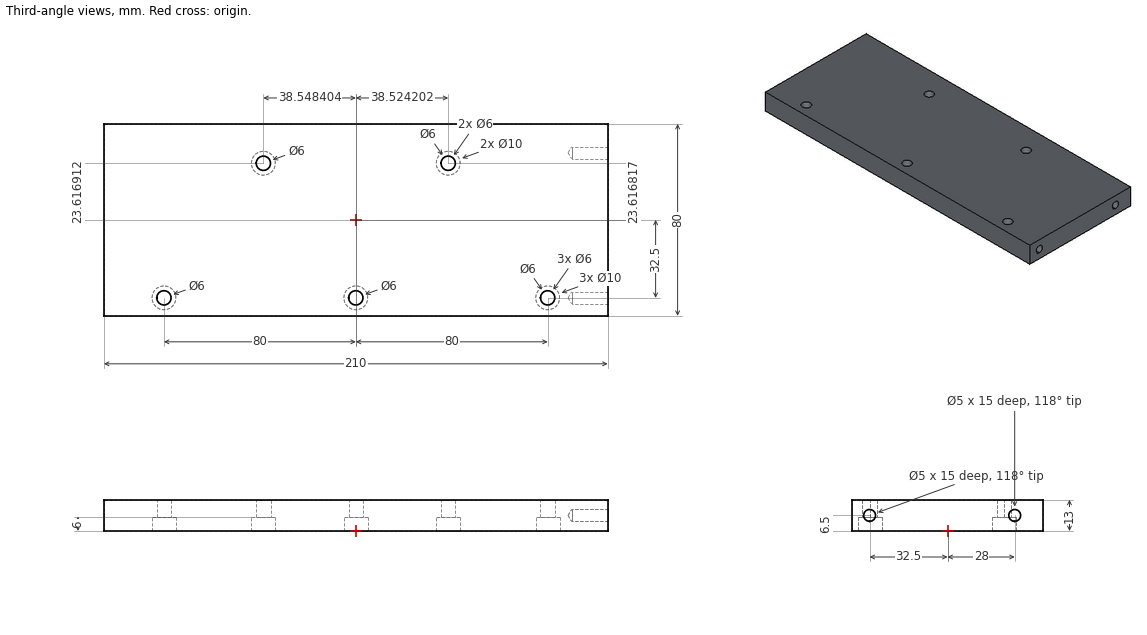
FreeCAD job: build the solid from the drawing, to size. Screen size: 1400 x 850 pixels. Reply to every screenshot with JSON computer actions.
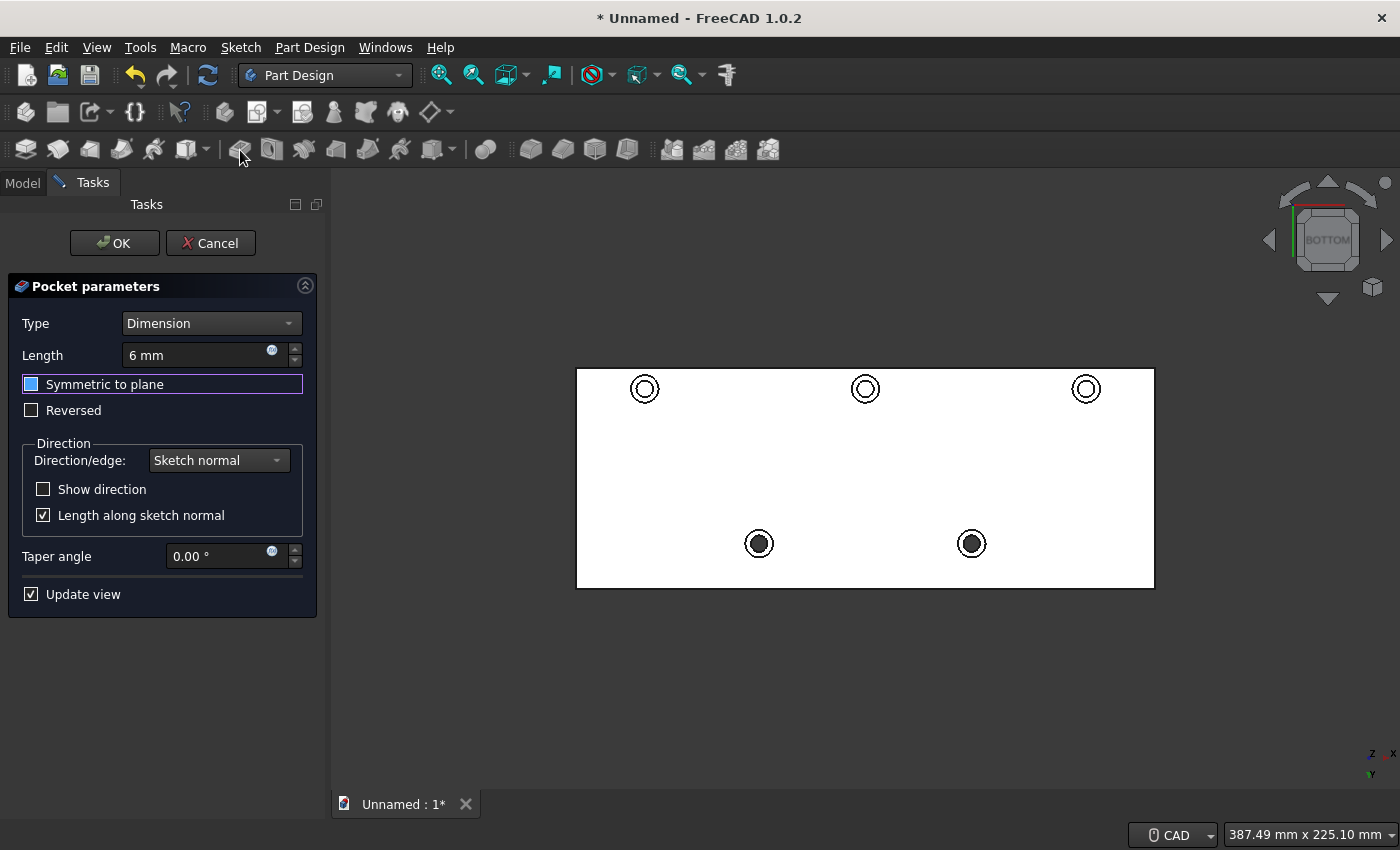
{"action": "left_click", "coordinate": [115, 243]}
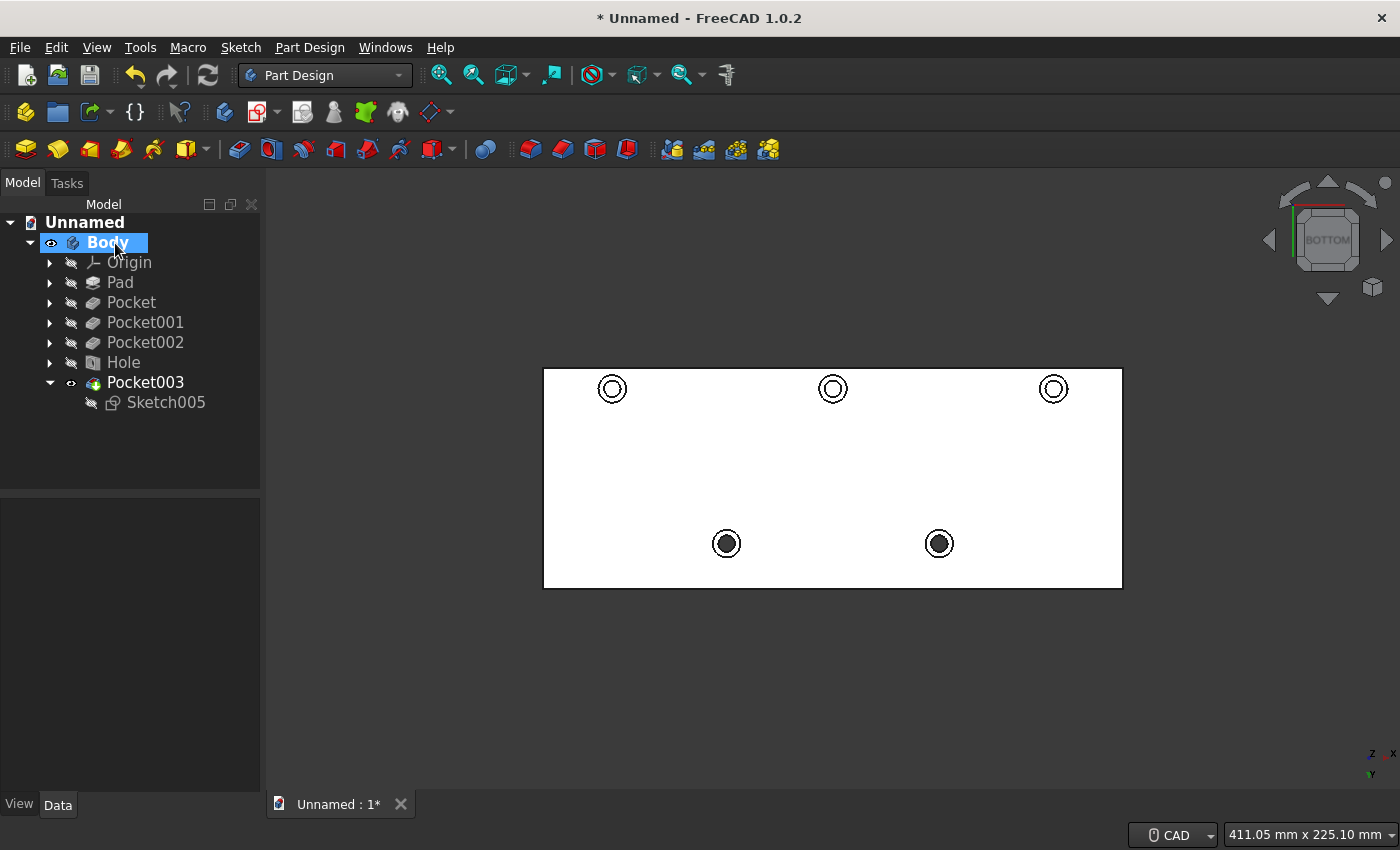
{"action": "left_click", "coordinate": [916, 446]}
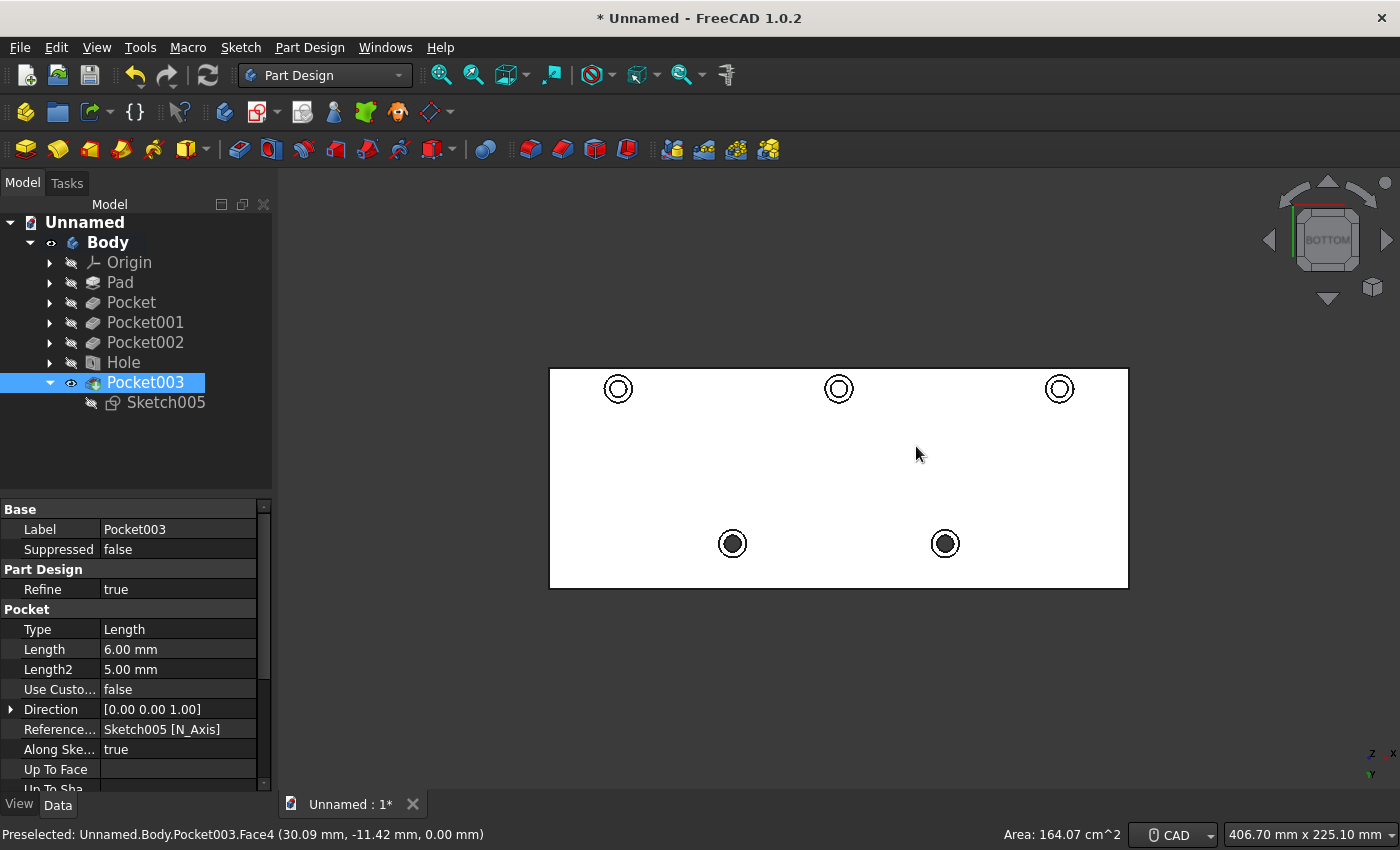
{"action": "left_click", "coordinate": [258, 112]}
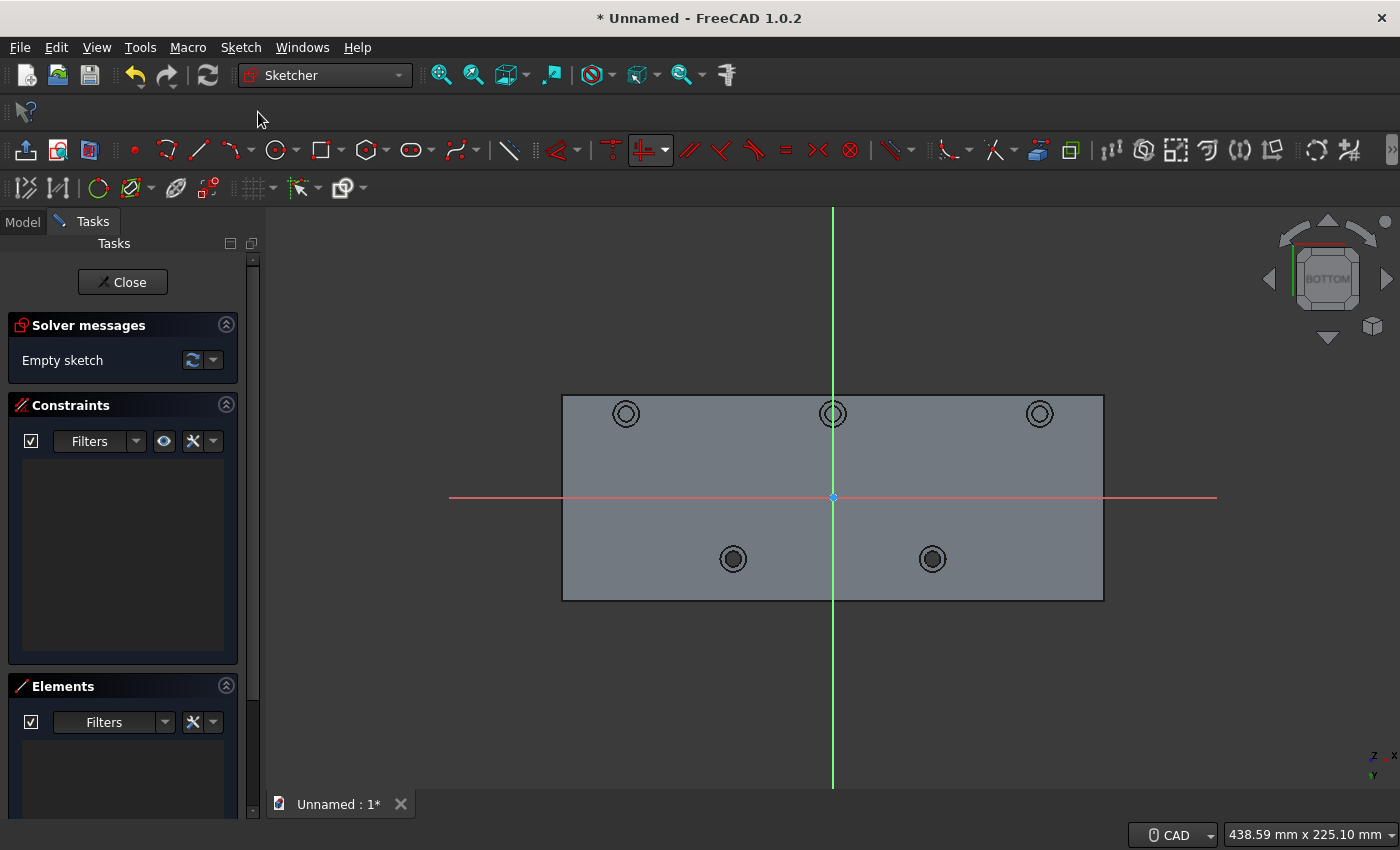
{"action": "scroll", "coordinate": [1054, 410], "scroll_direction": "up", "scroll_amount": 15}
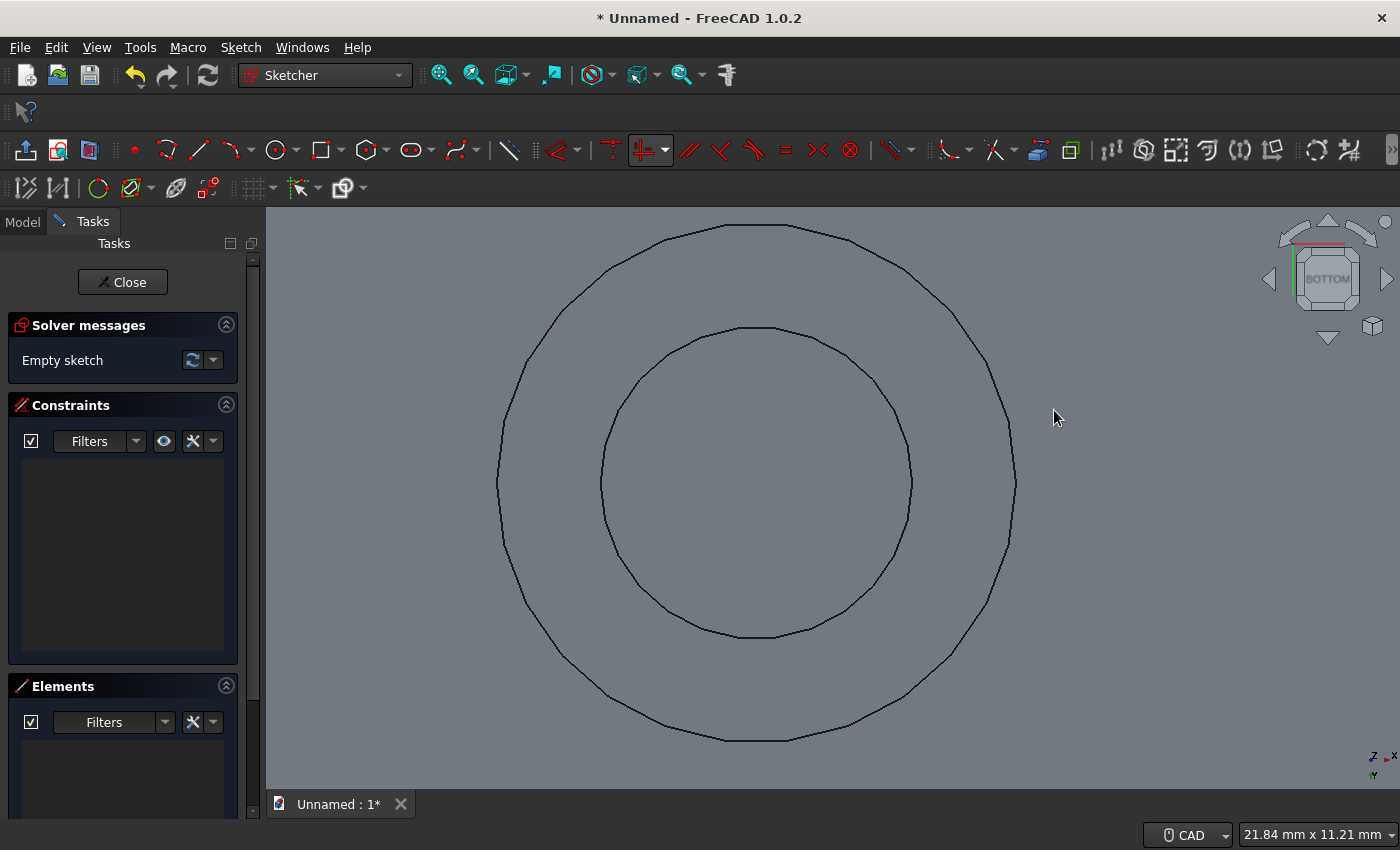
{"action": "key", "text": "g c"}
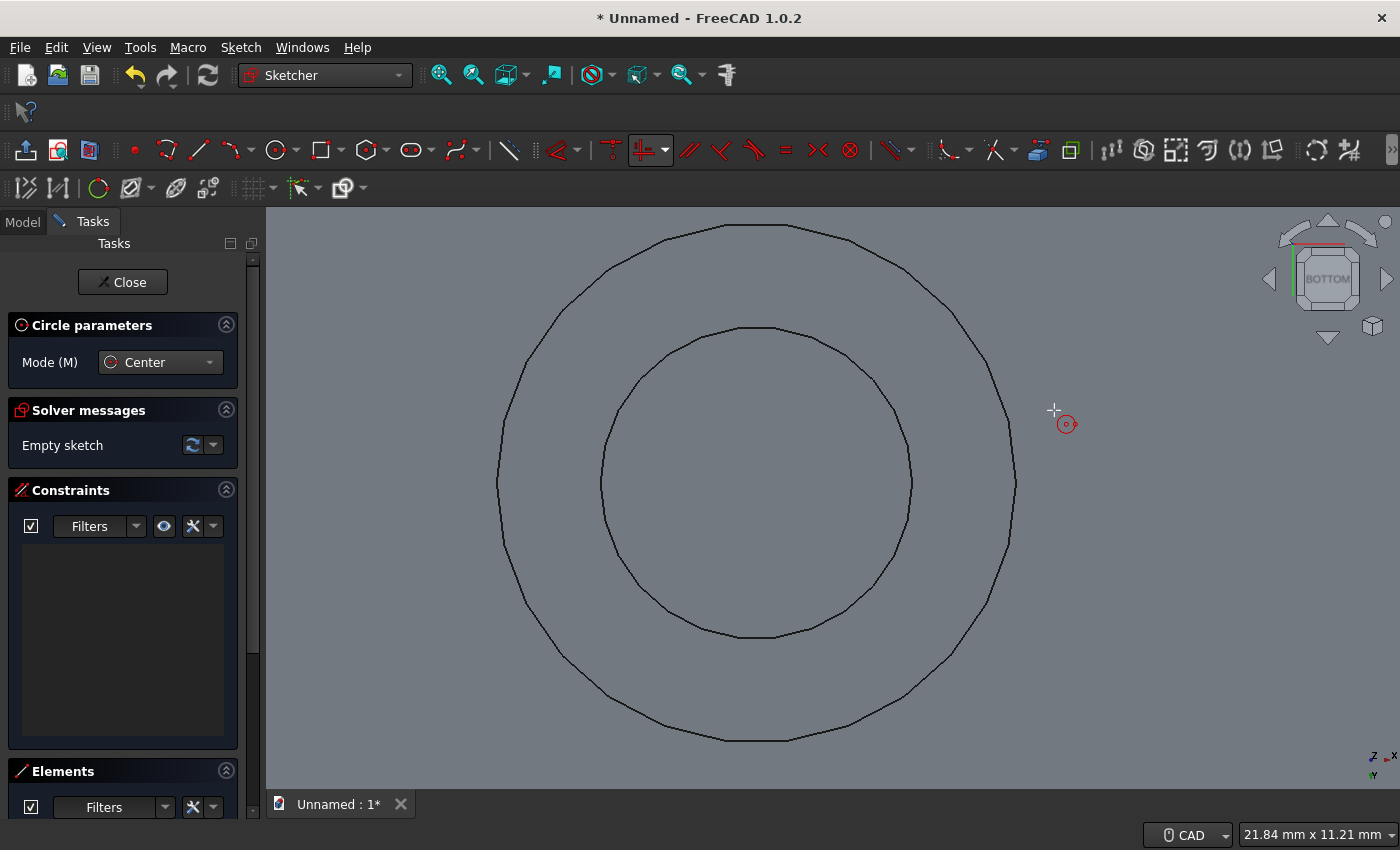
{"action": "left_click", "coordinate": [756, 483]}
{"action": "left_click", "coordinate": [867, 373]}
{"action": "key", "text": "Escape"}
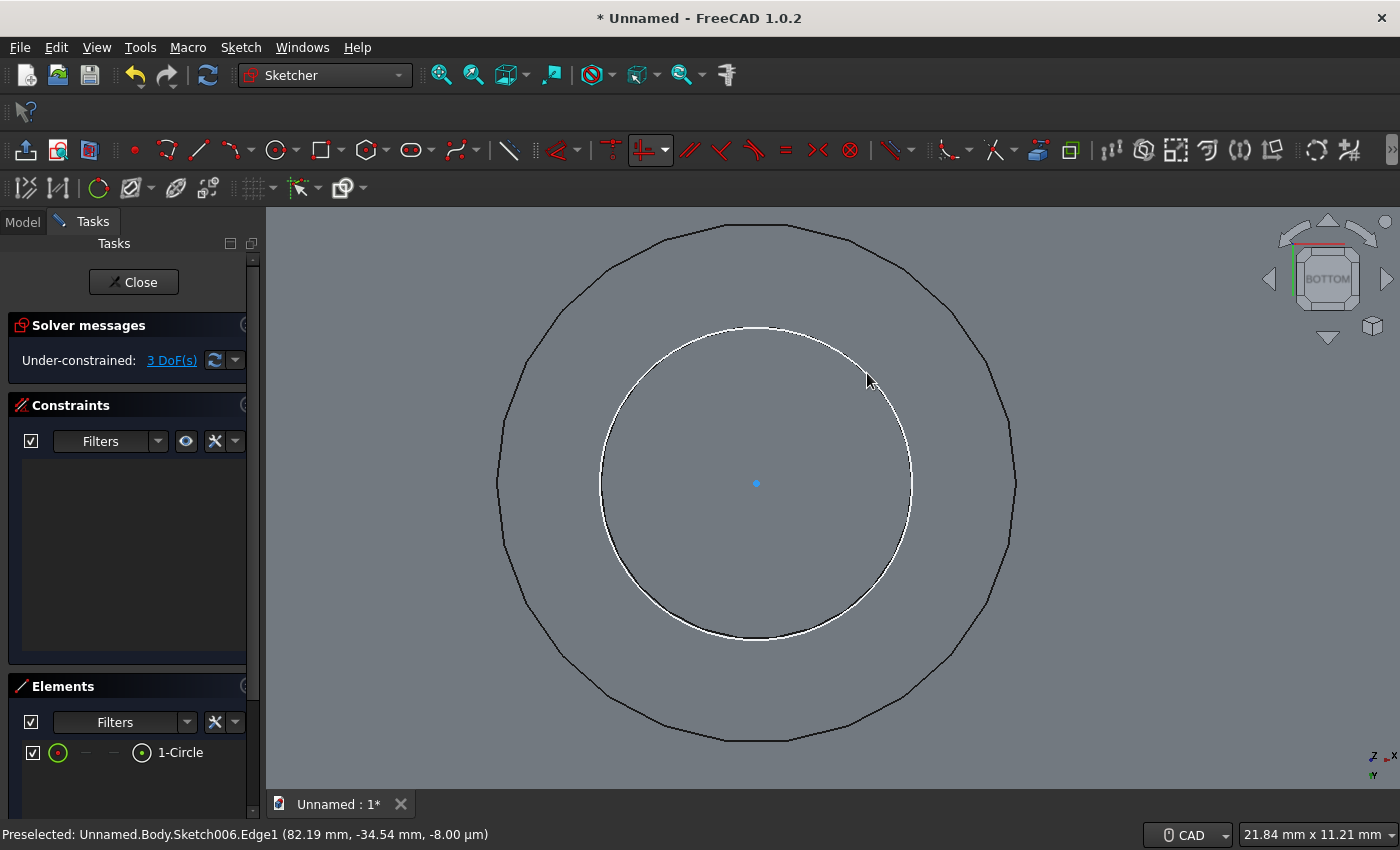
{"action": "key", "text": "d"}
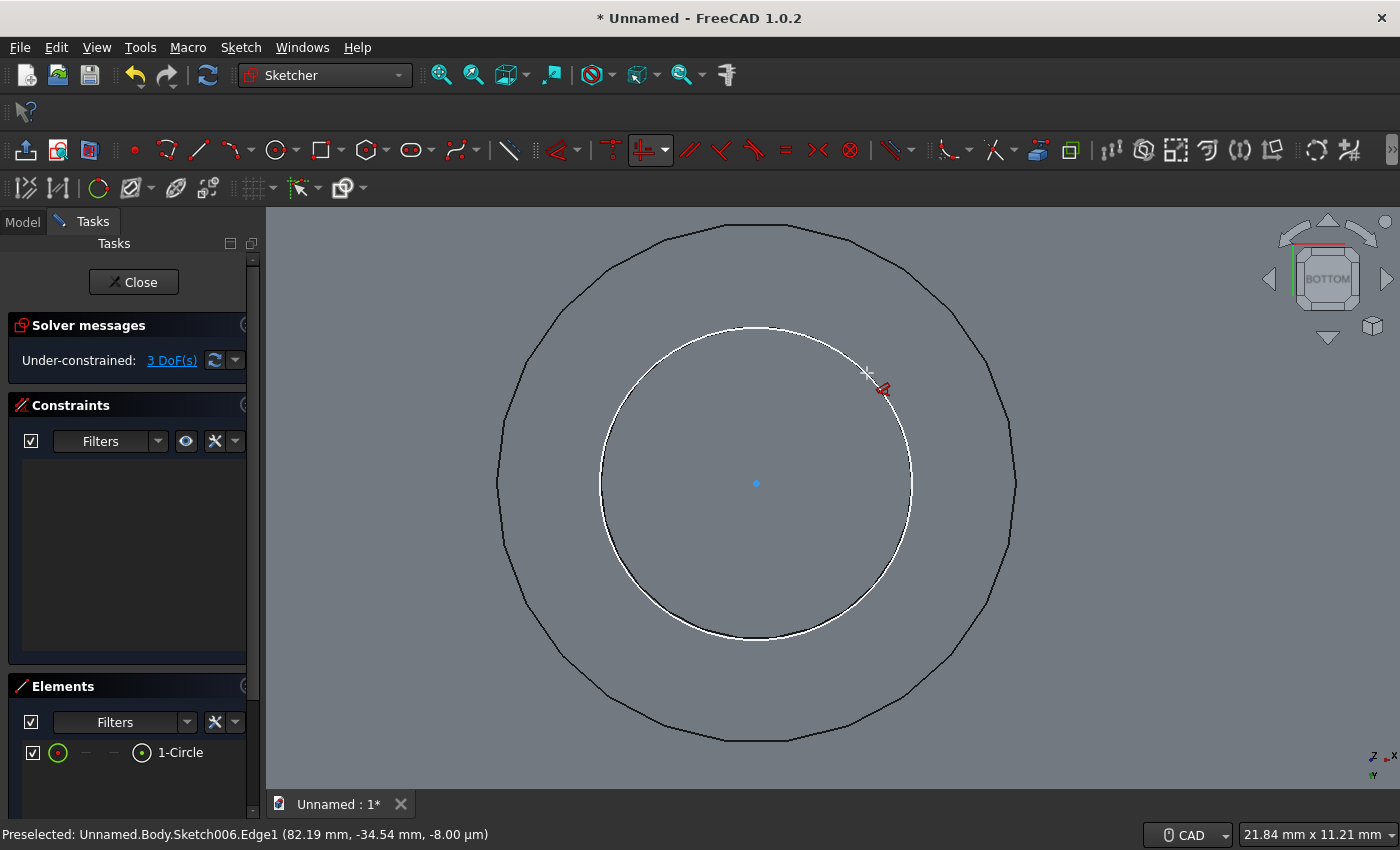
{"action": "left_click", "coordinate": [866, 373]}
{"action": "left_click", "coordinate": [889, 350]}